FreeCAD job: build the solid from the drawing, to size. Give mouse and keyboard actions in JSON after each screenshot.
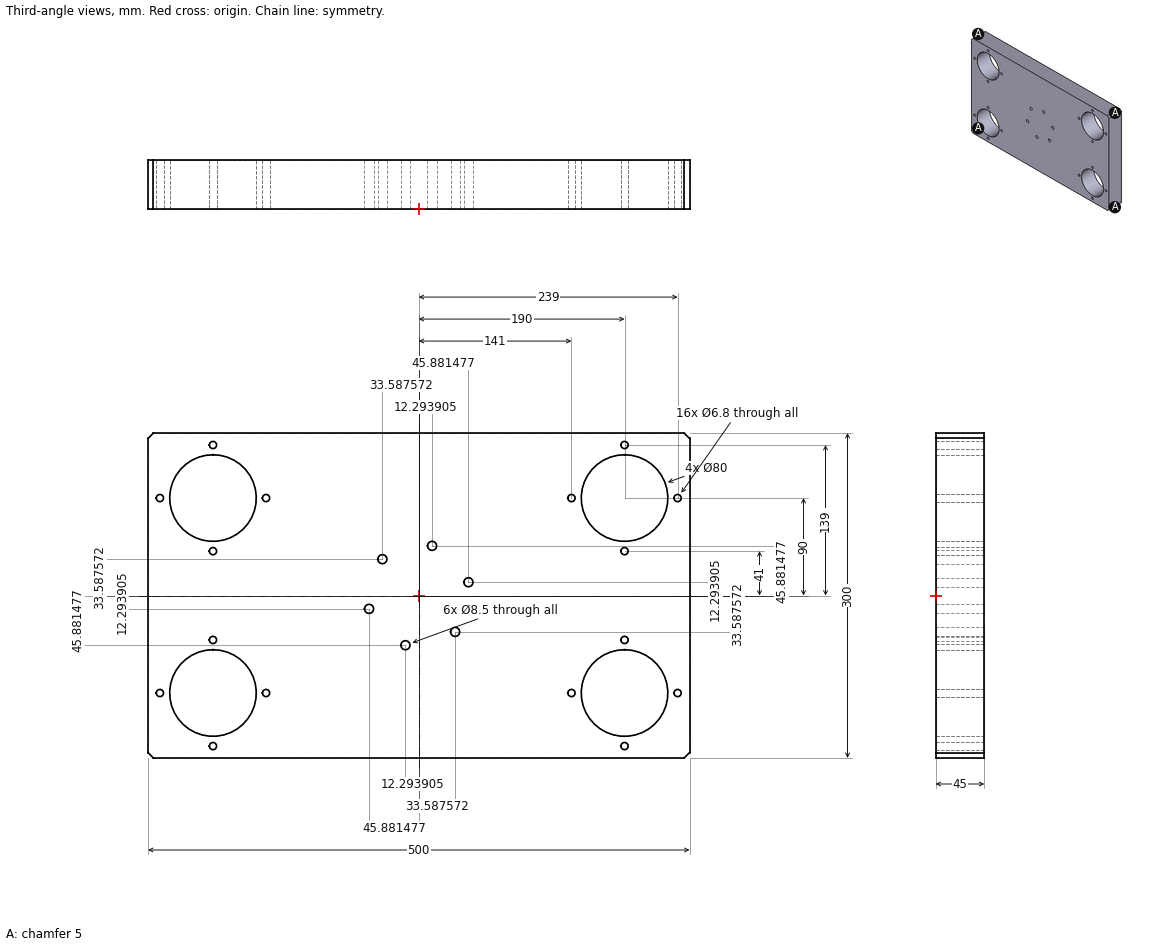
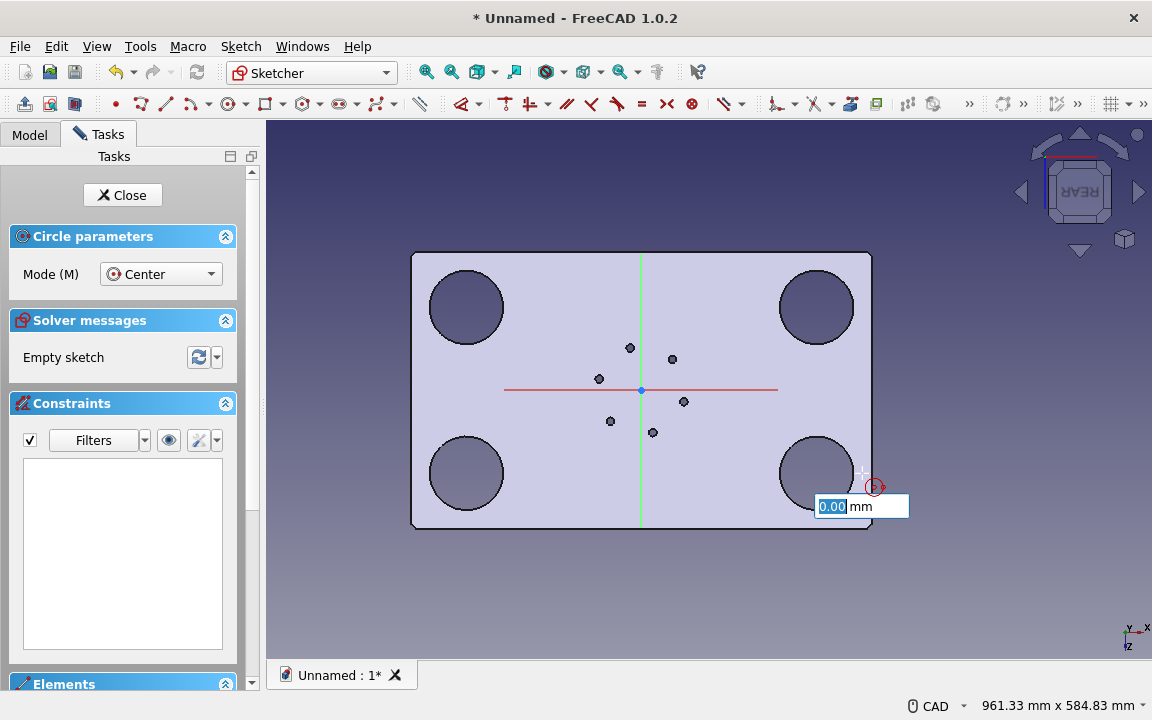
{"action": "scroll", "coordinate": [864, 471], "scroll_direction": "up", "scroll_amount": 9}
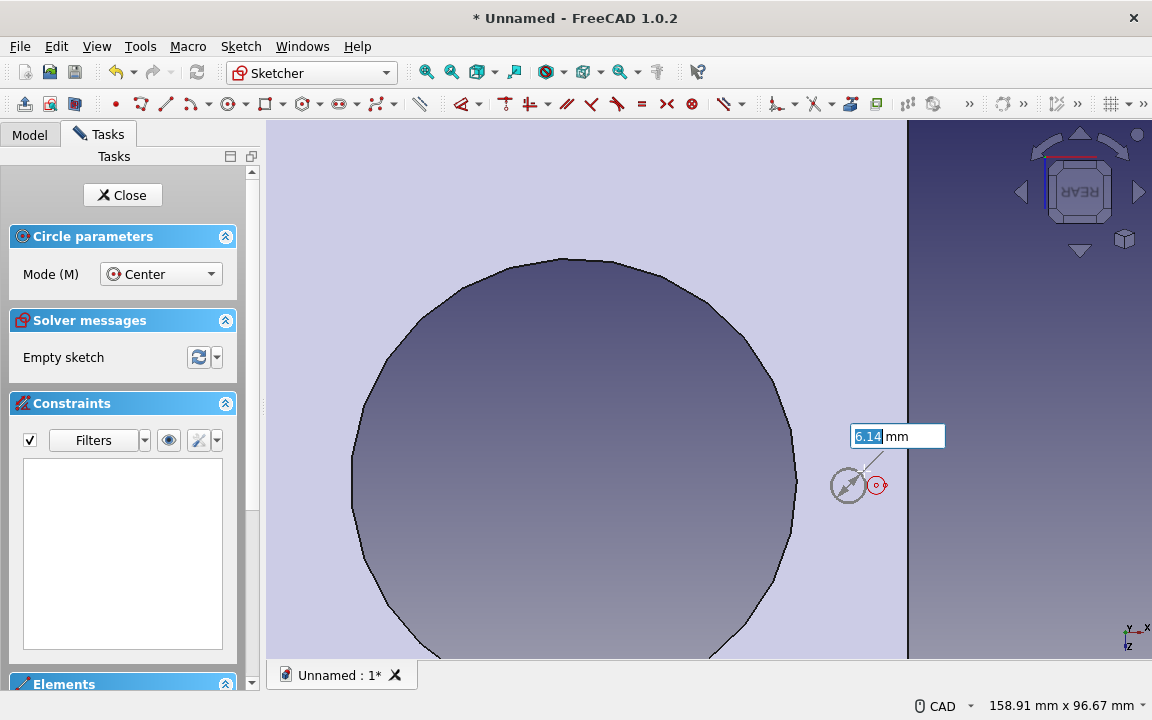
{"action": "left_click", "coordinate": [860, 468]}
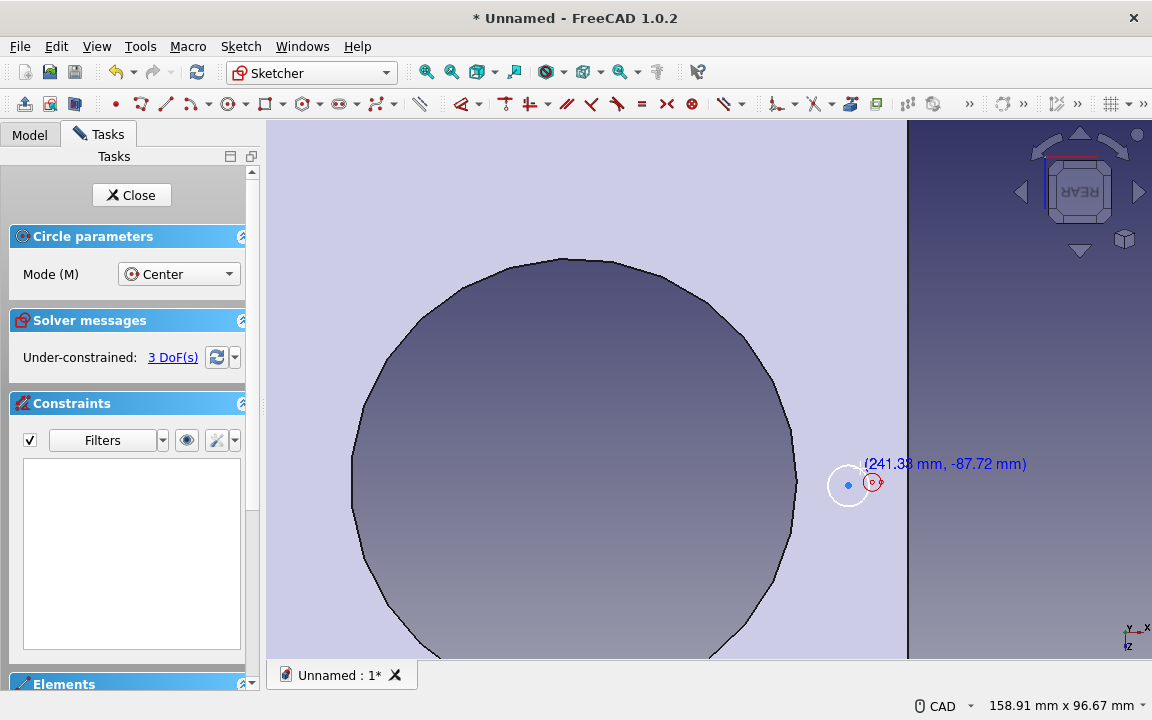
{"action": "scroll", "coordinate": [864, 471], "scroll_direction": "down", "scroll_amount": 9}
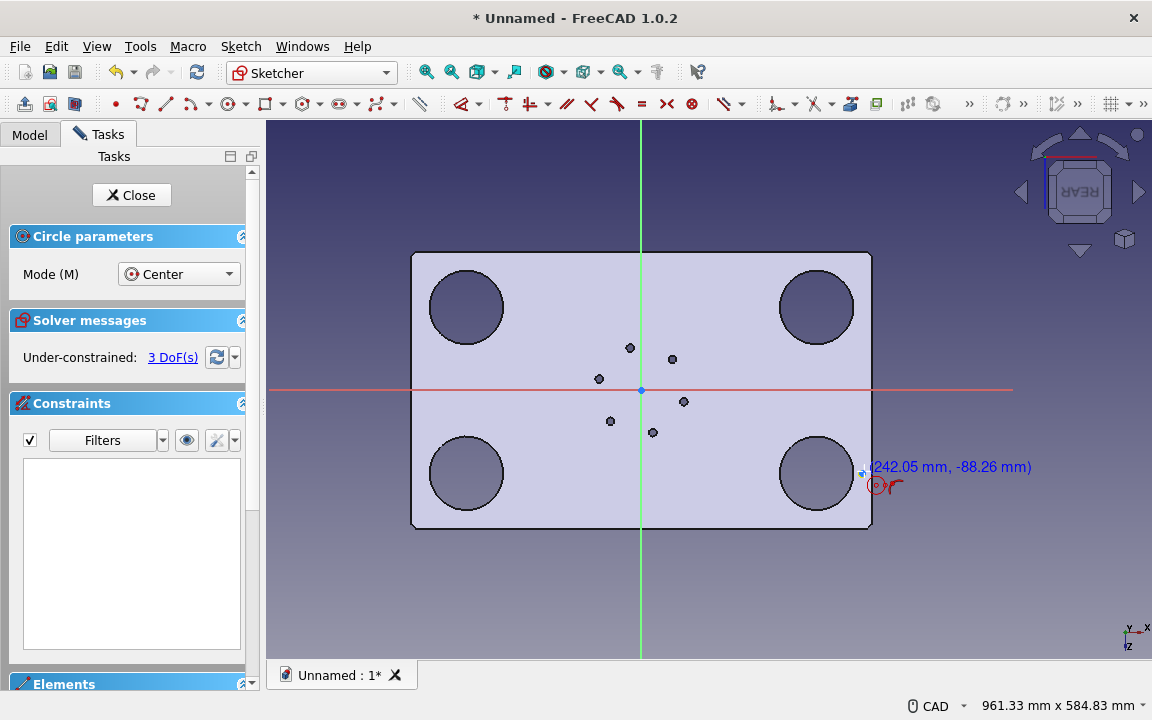
{"action": "scroll", "coordinate": [817, 518], "scroll_direction": "up", "scroll_amount": 10}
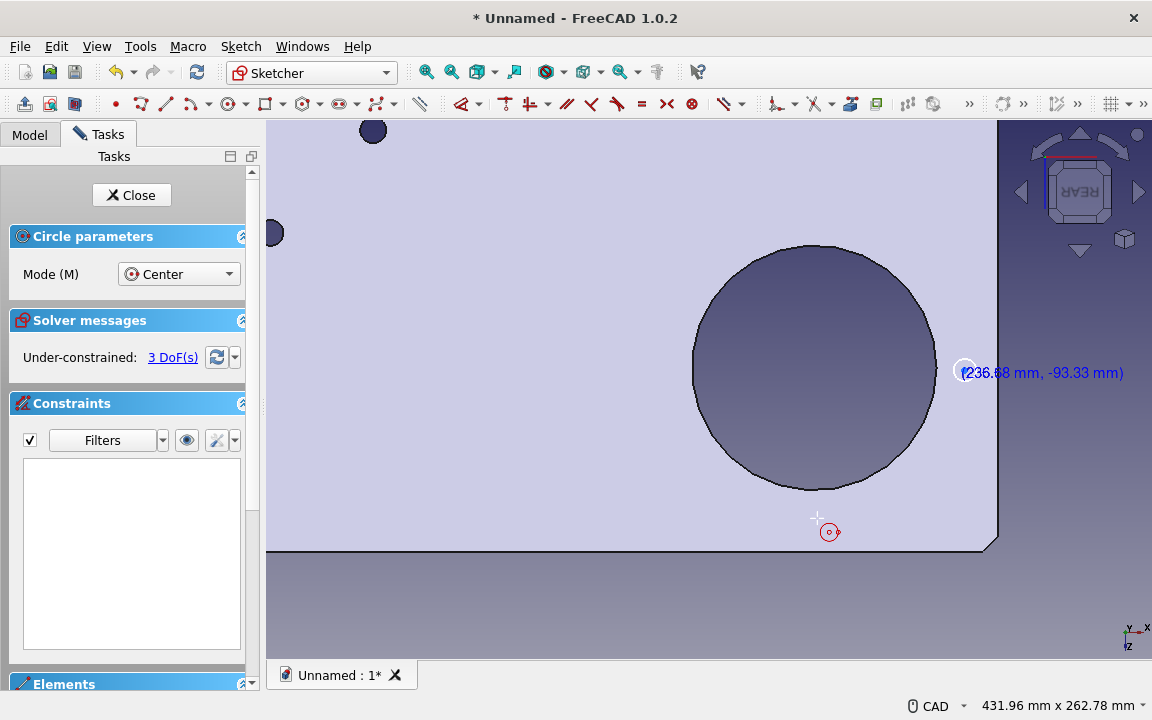
{"action": "scroll", "coordinate": [816, 518], "scroll_direction": "down", "scroll_amount": 10}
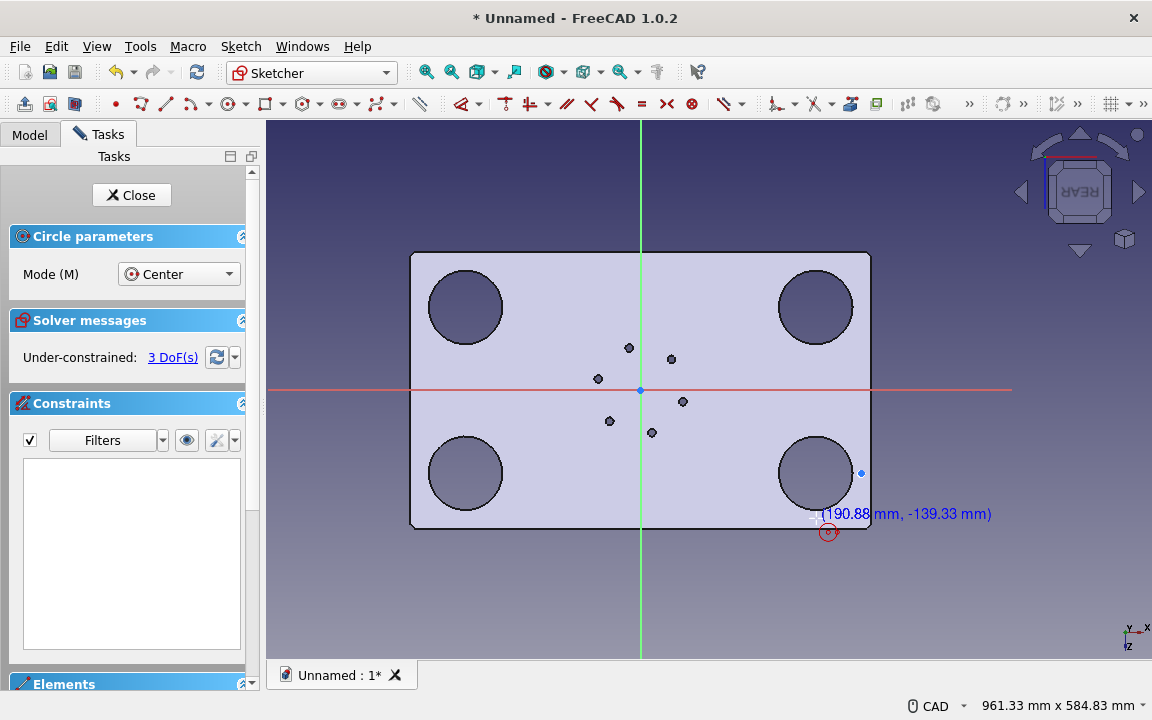
{"action": "left_click", "coordinate": [816, 518]}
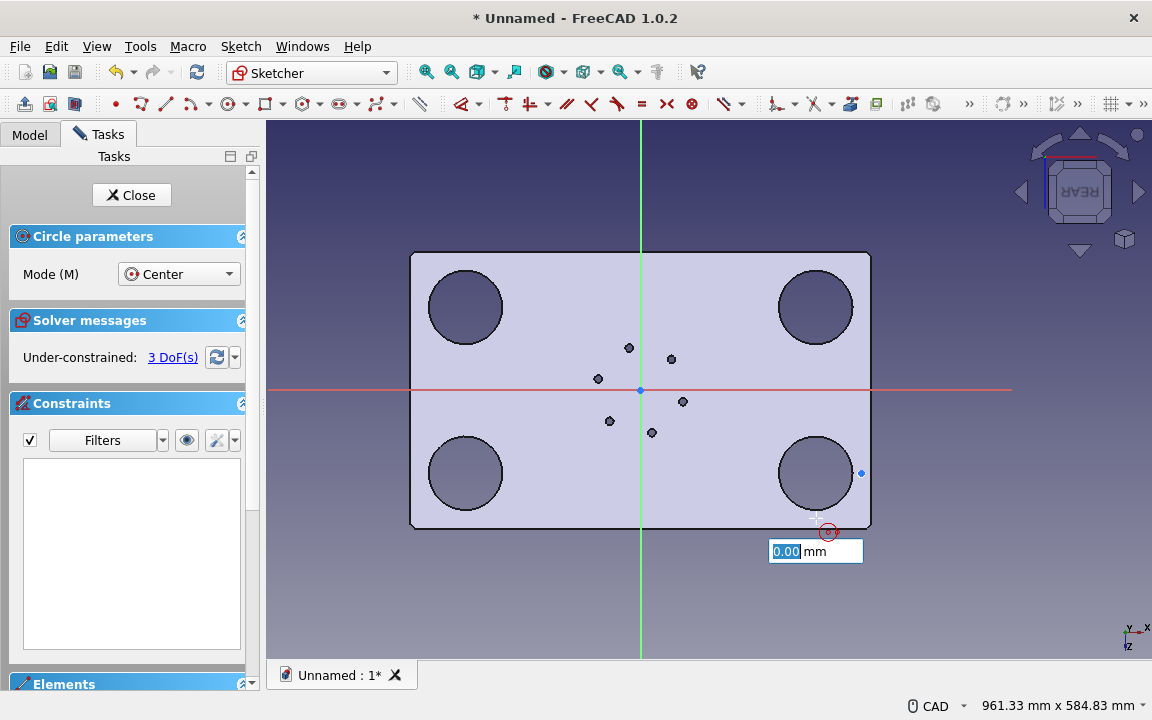
{"action": "scroll", "coordinate": [818, 516], "scroll_direction": "up", "scroll_amount": 9}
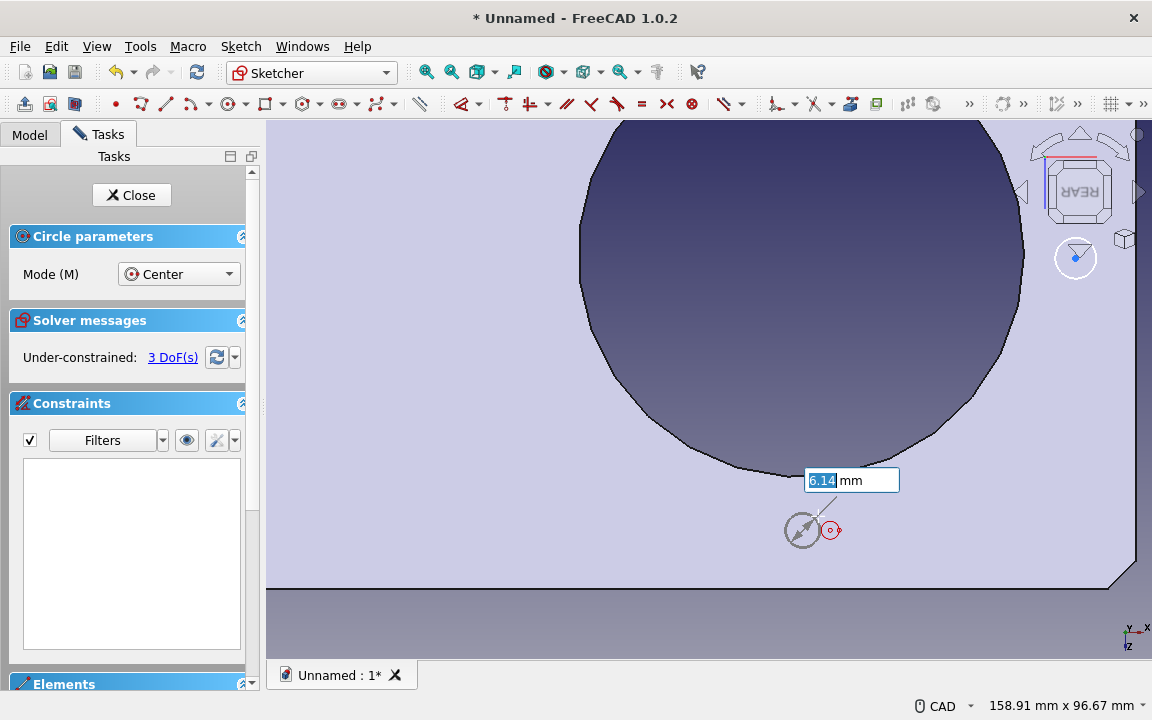
{"action": "left_click", "coordinate": [814, 514]}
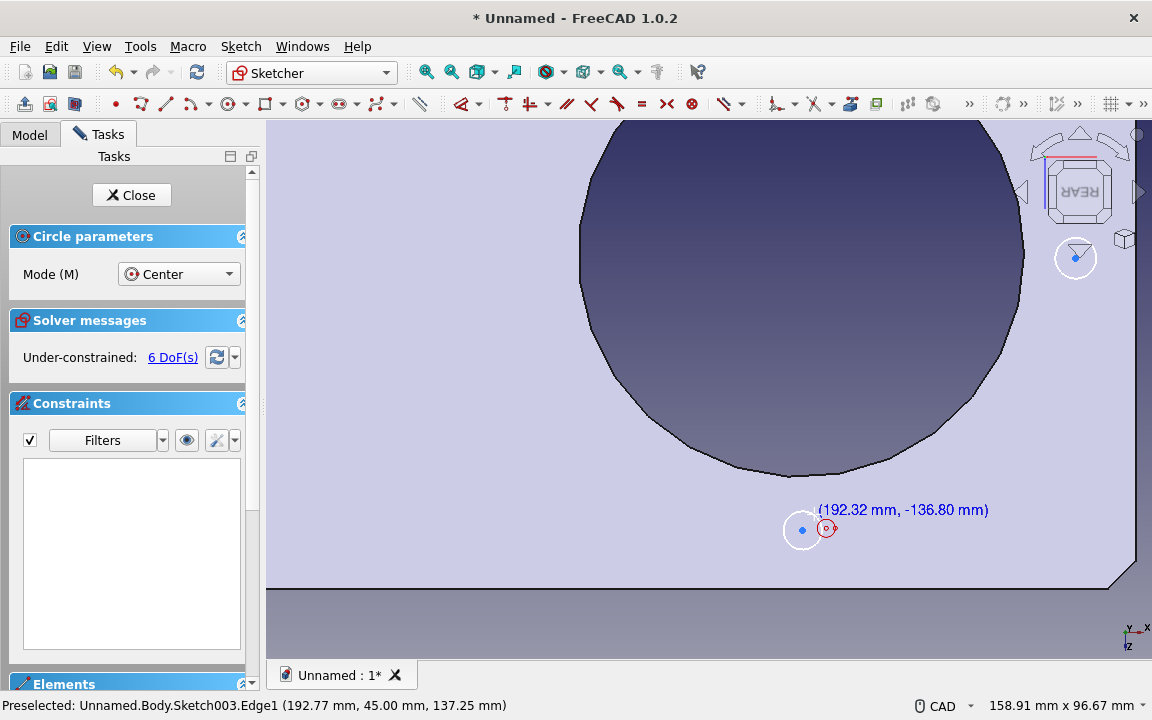
{"action": "scroll", "coordinate": [818, 516], "scroll_direction": "down", "scroll_amount": 9}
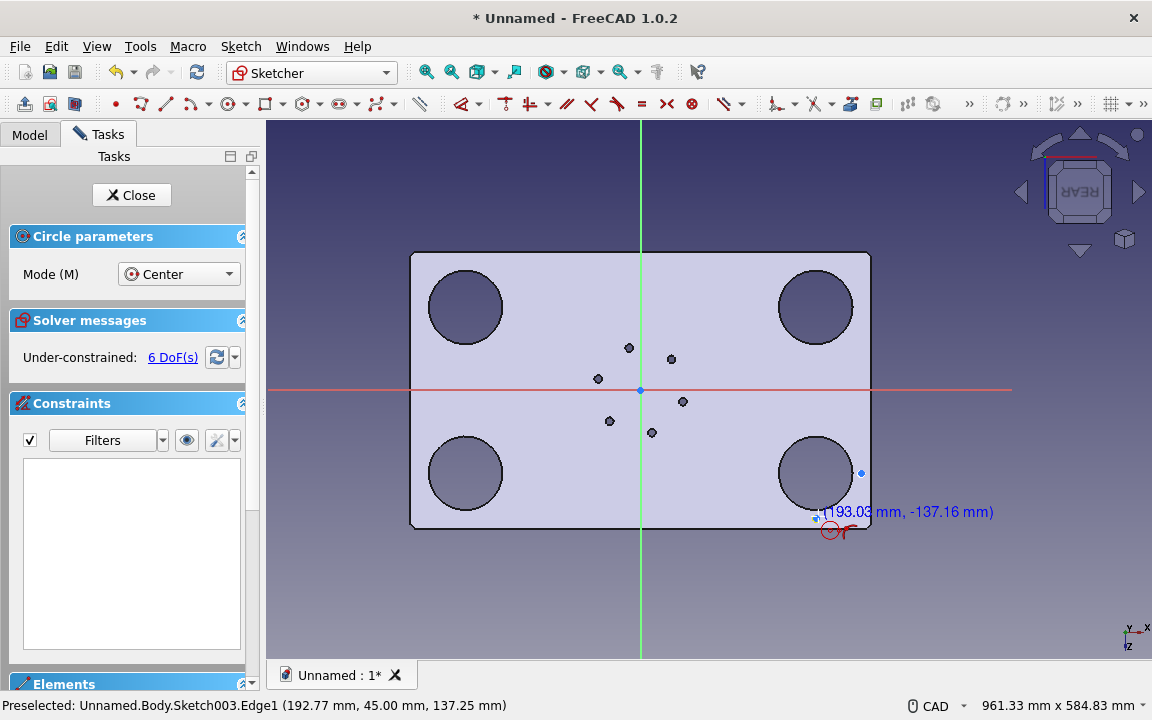
{"action": "left_click", "coordinate": [771, 473]}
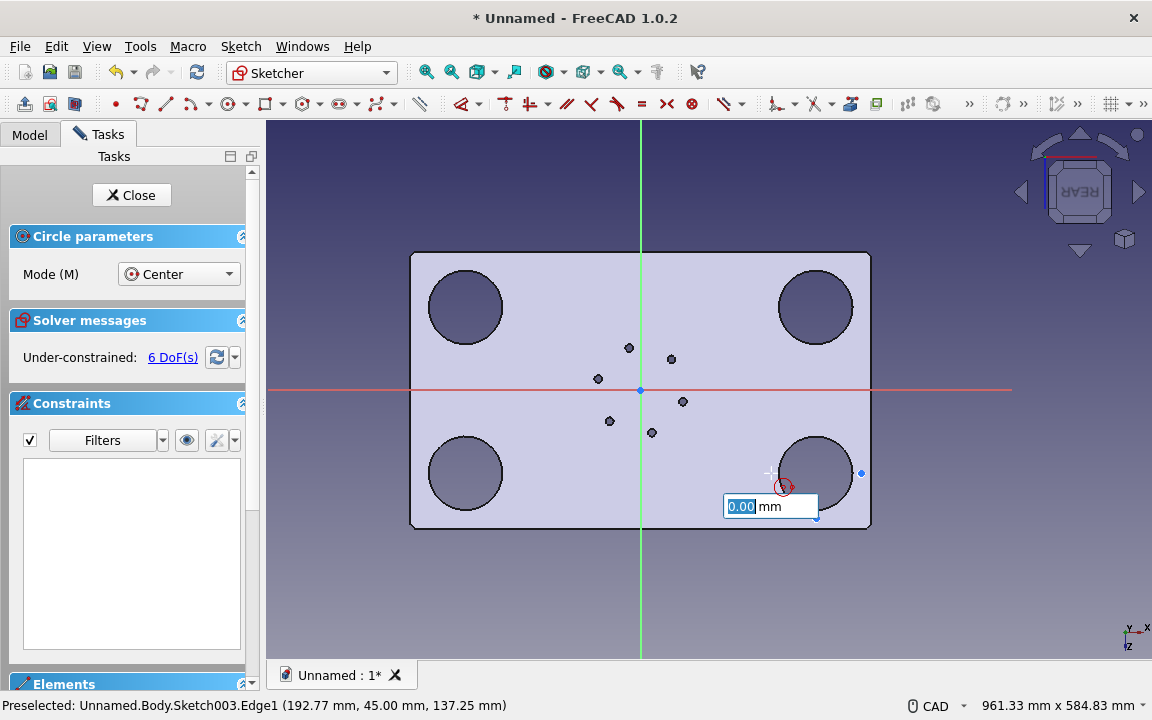
{"action": "scroll", "coordinate": [773, 471], "scroll_direction": "up", "scroll_amount": 9}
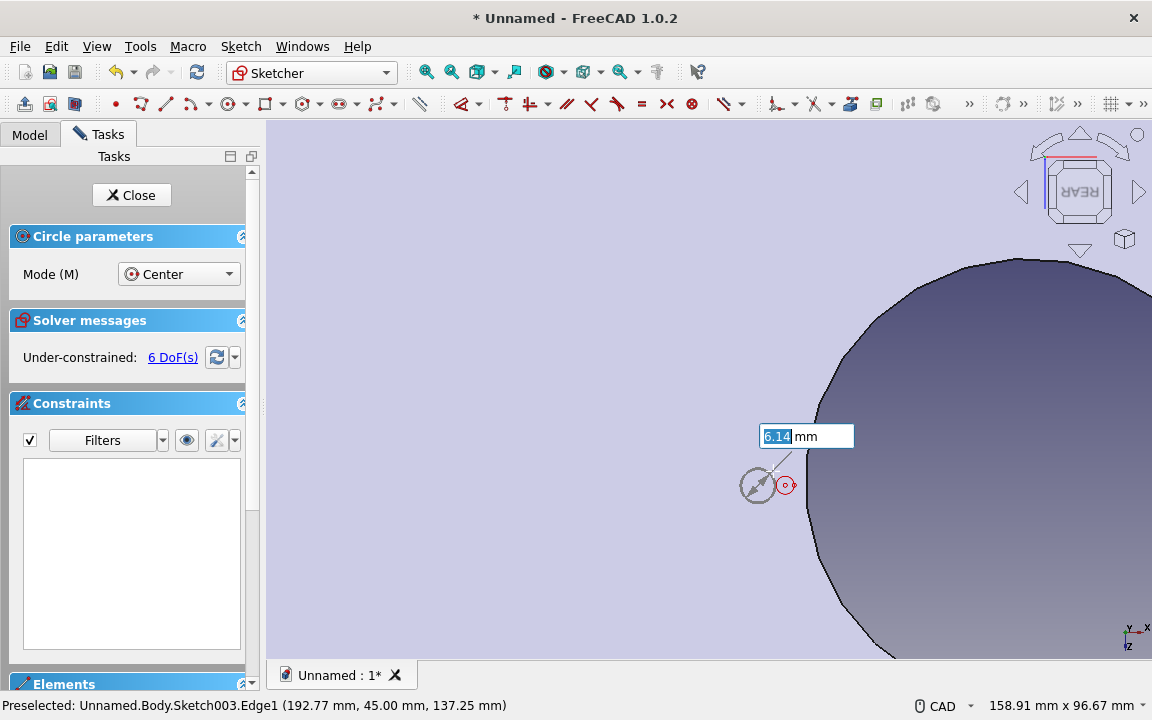
{"action": "left_click", "coordinate": [769, 468]}